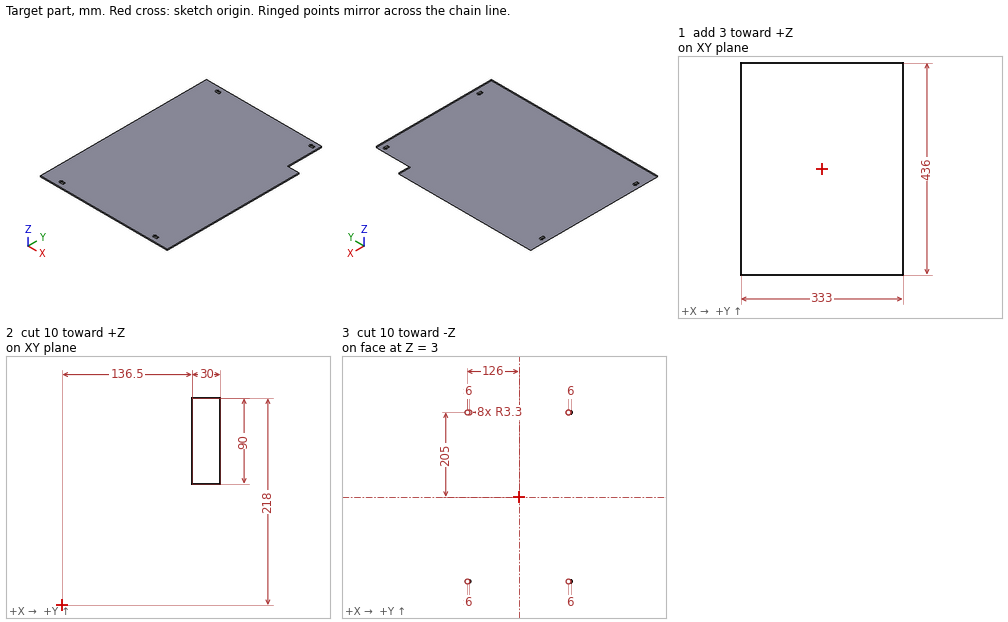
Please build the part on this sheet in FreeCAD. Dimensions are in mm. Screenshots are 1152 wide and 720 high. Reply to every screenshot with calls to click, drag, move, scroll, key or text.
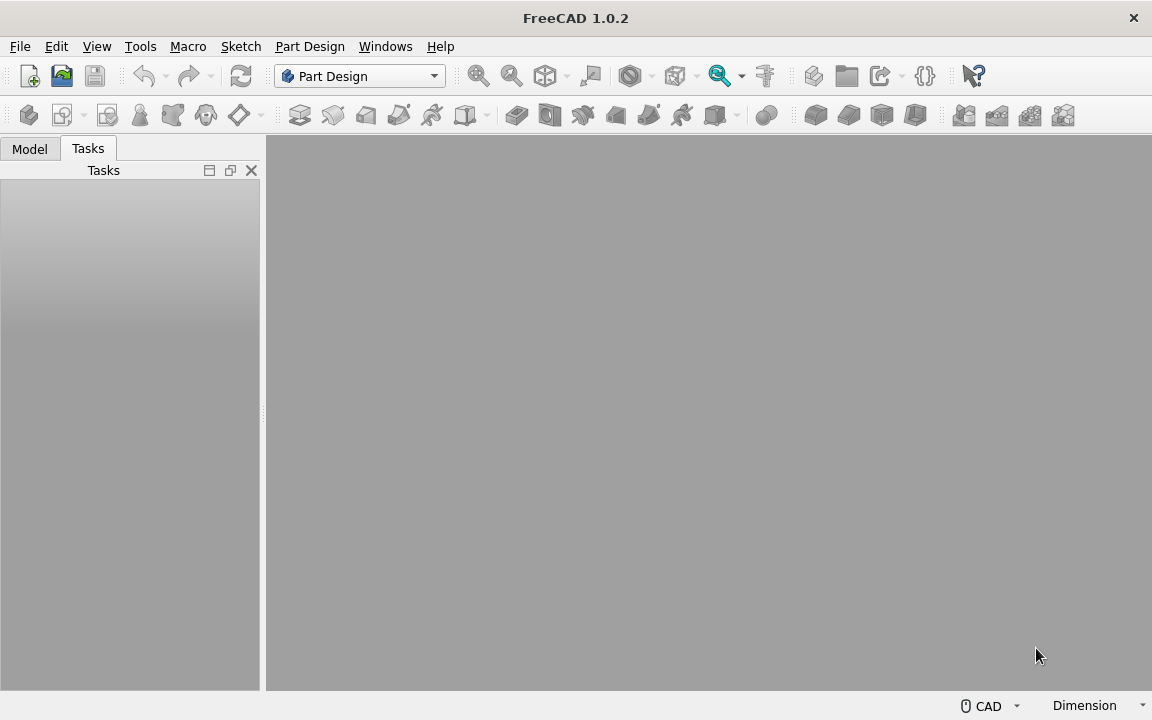
click(29, 76)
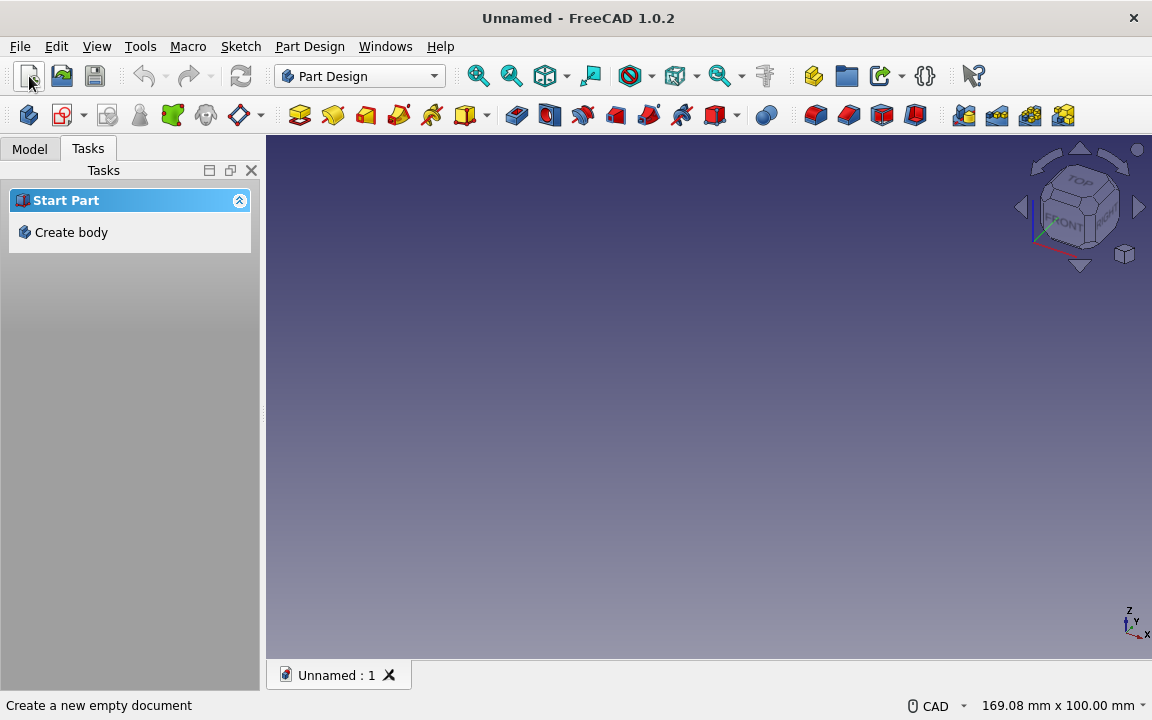
click(62, 116)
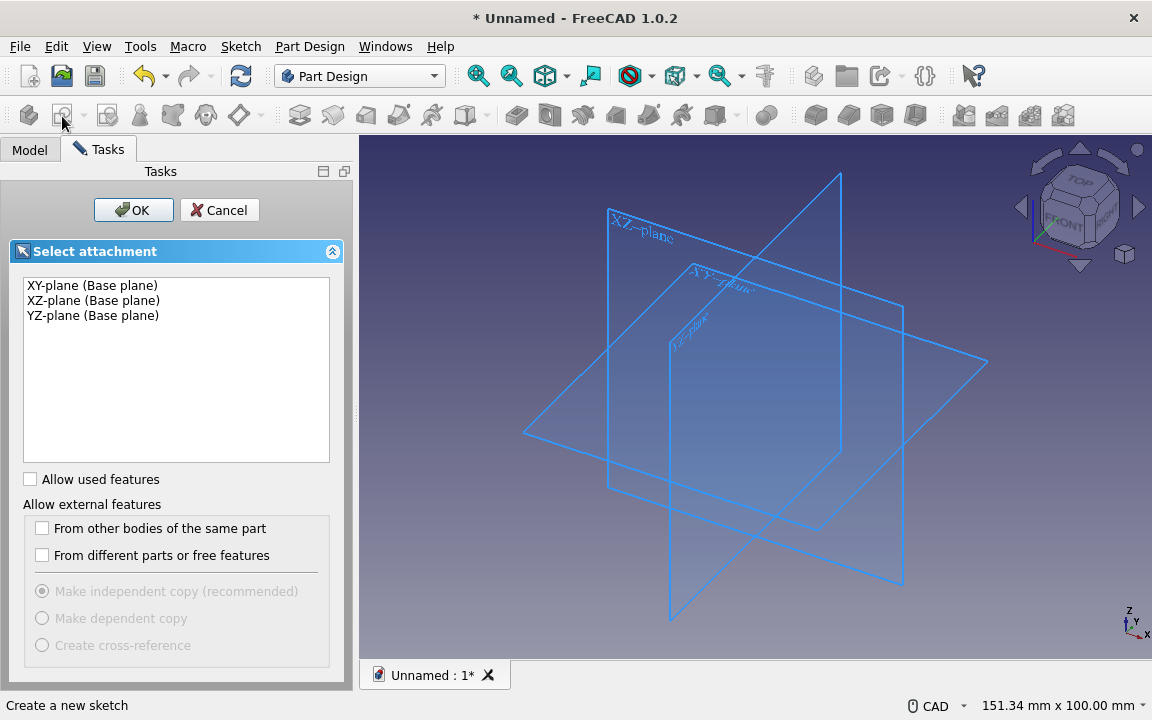
click(84, 286)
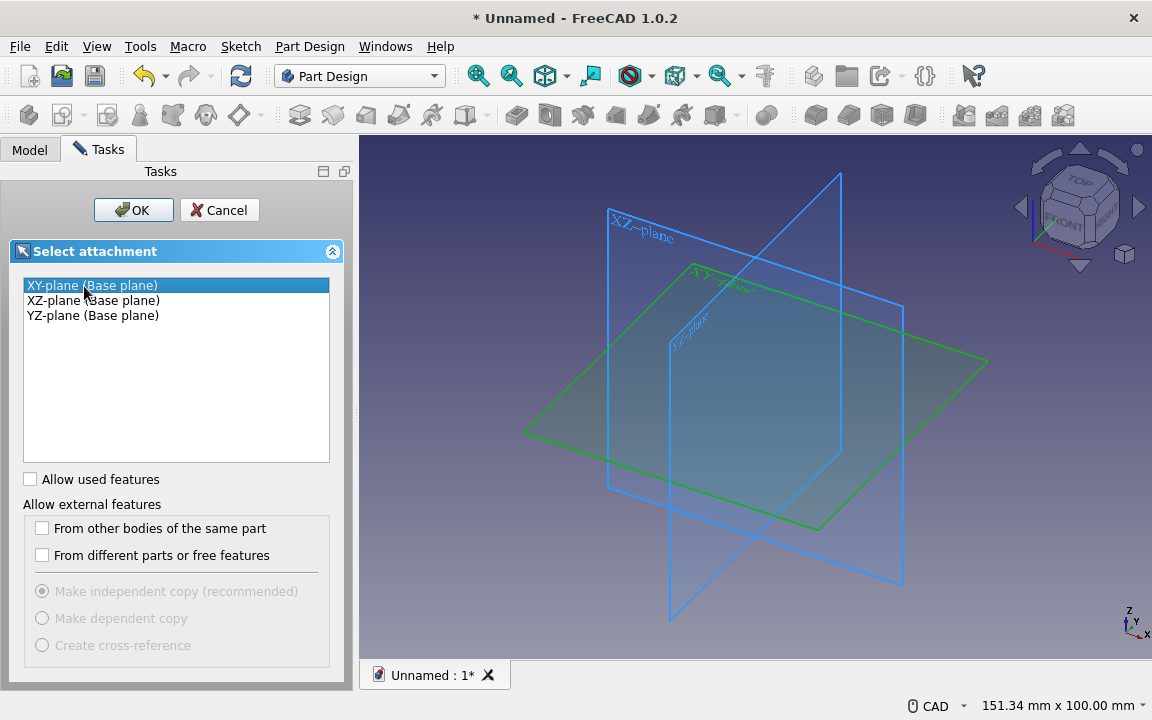
click(134, 210)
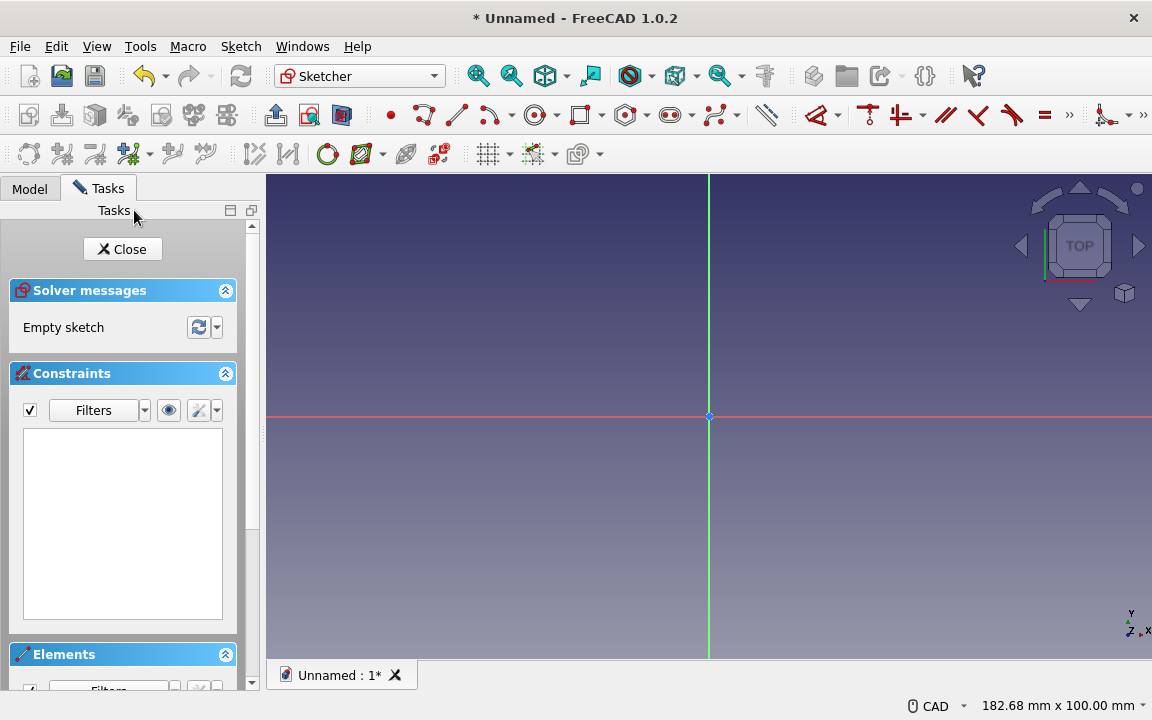
scroll(630, 416, down, 10)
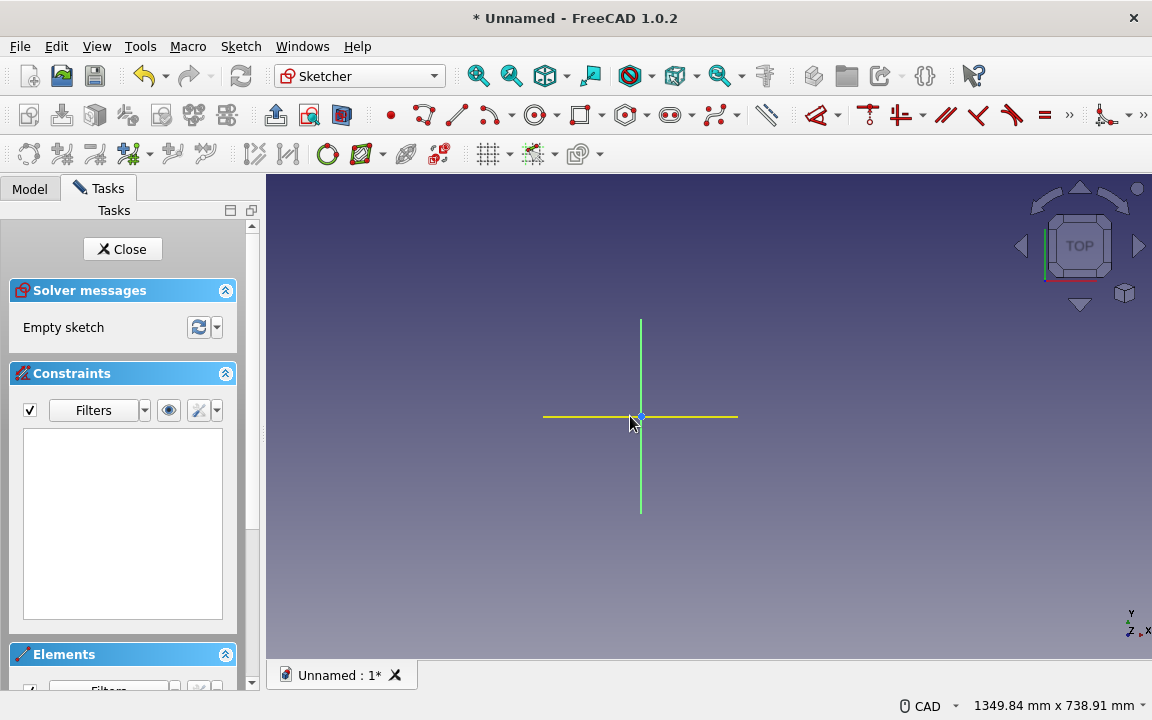
key(g)
key(v)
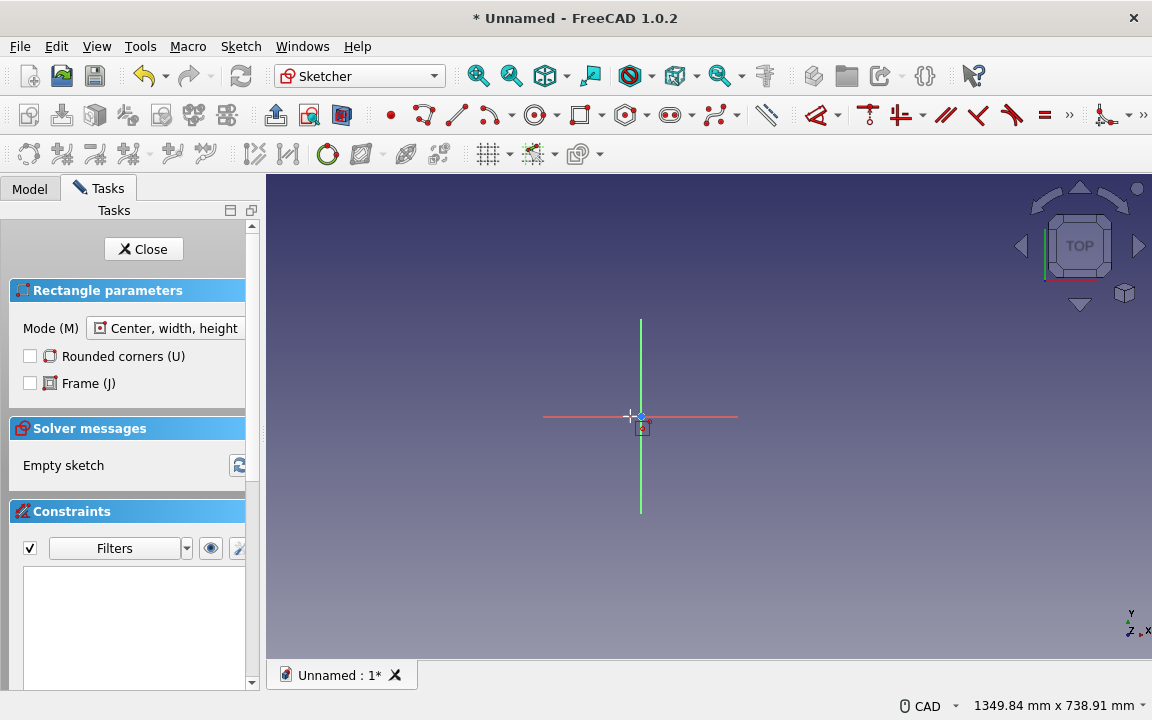
click(641, 416)
click(750, 273)
key(Escape)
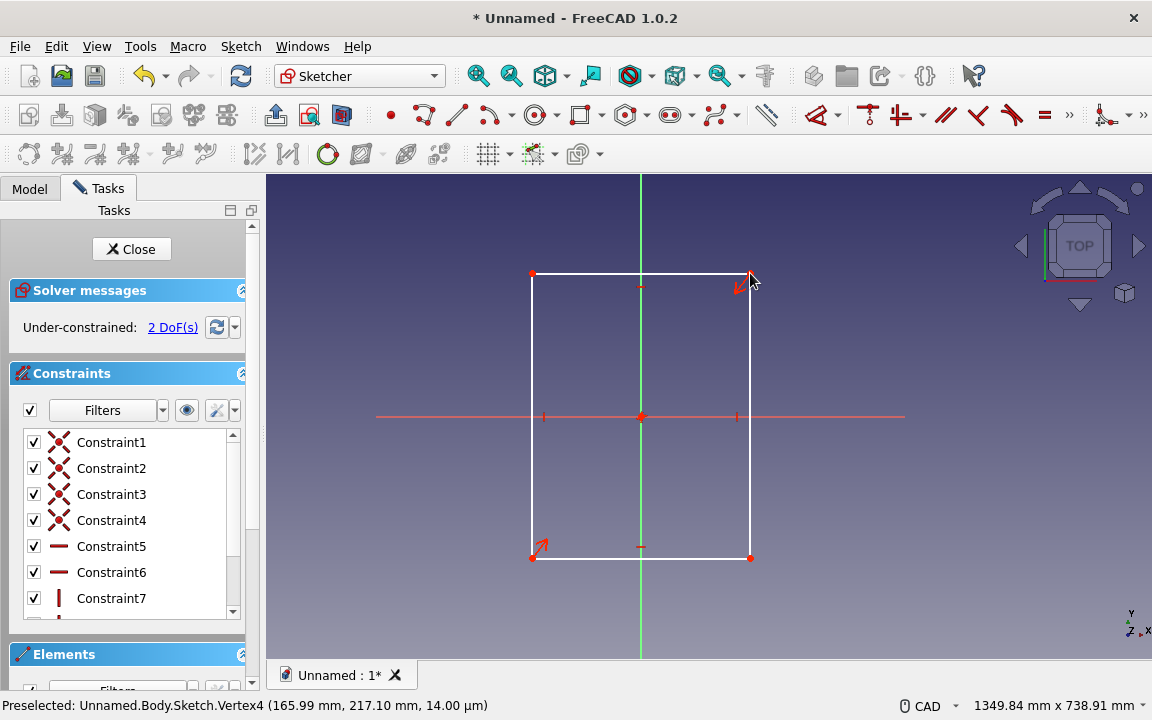
click(816, 116)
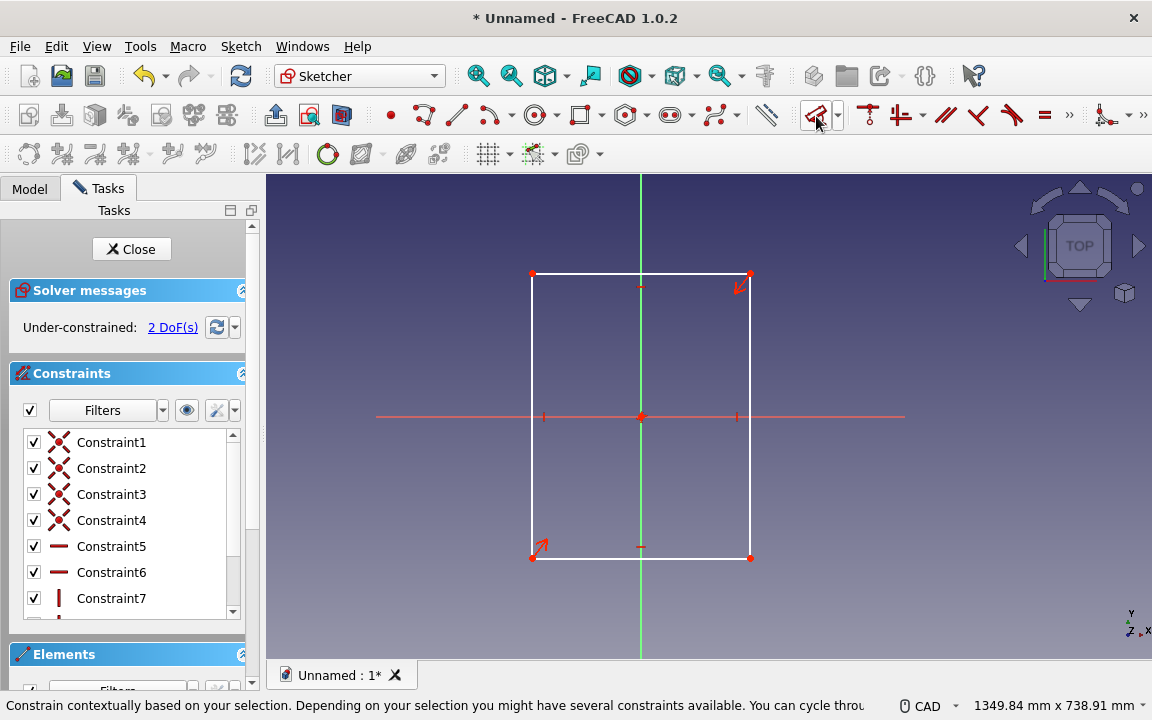
click(597, 559)
click(591, 593)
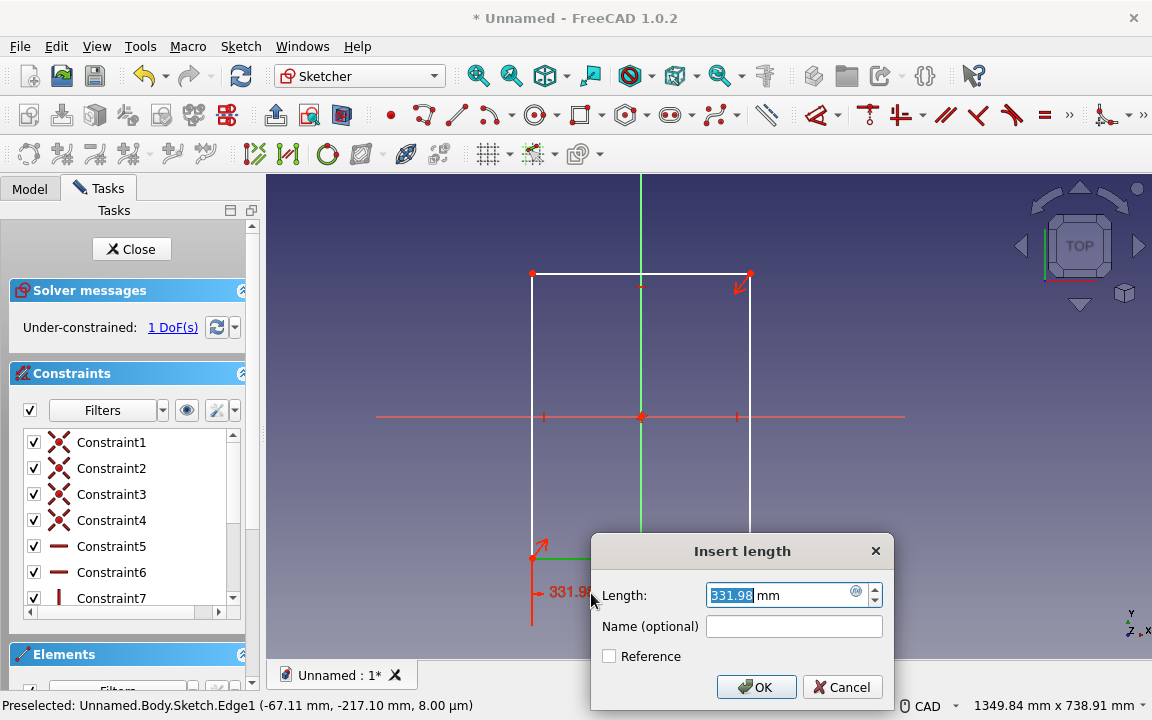
text(333)
key(Return)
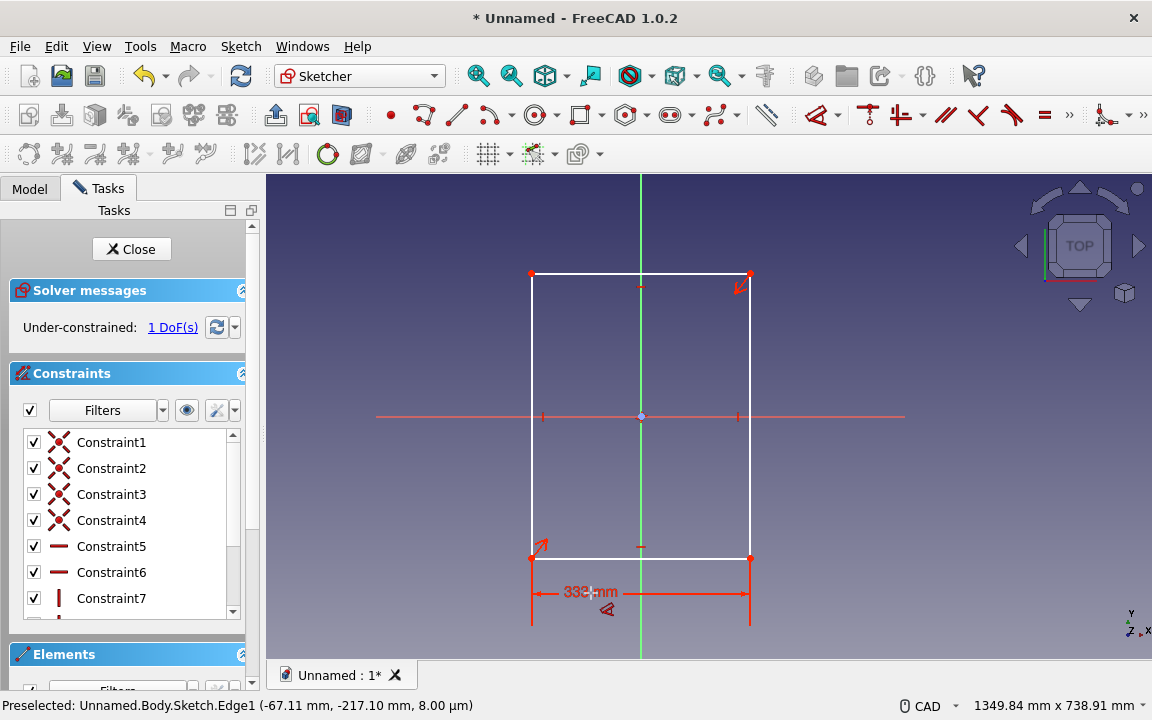
click(750, 473)
click(784, 351)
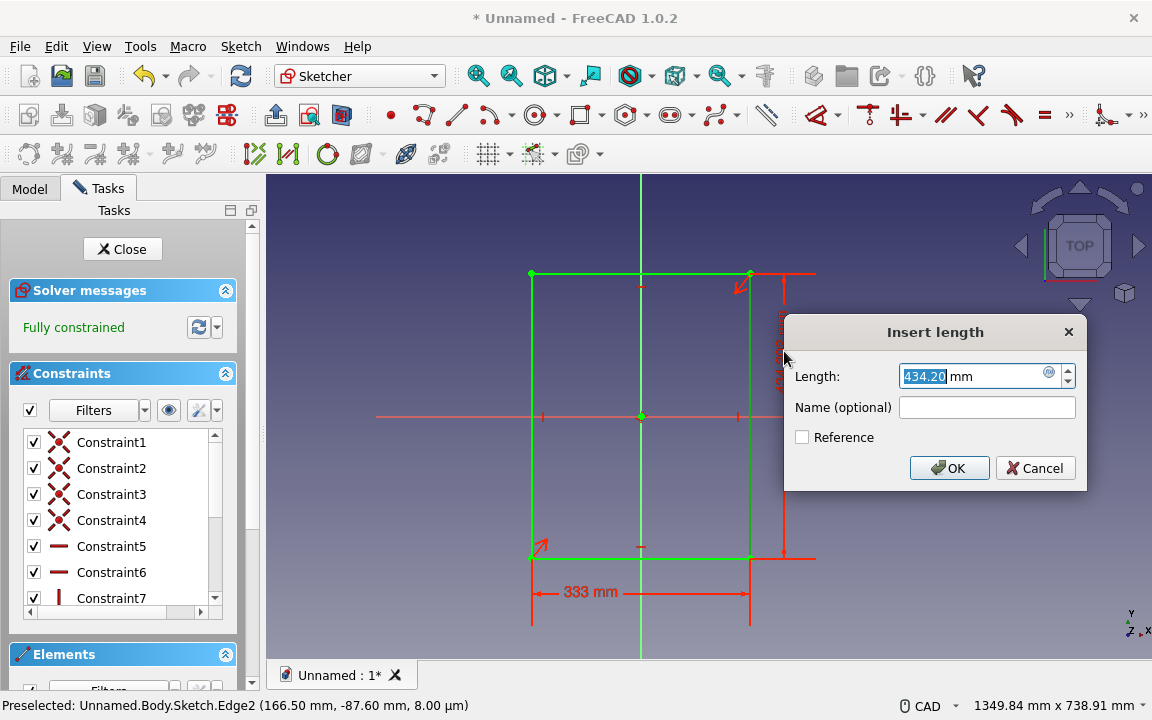
text(436)
key(Return)
key(Escape)